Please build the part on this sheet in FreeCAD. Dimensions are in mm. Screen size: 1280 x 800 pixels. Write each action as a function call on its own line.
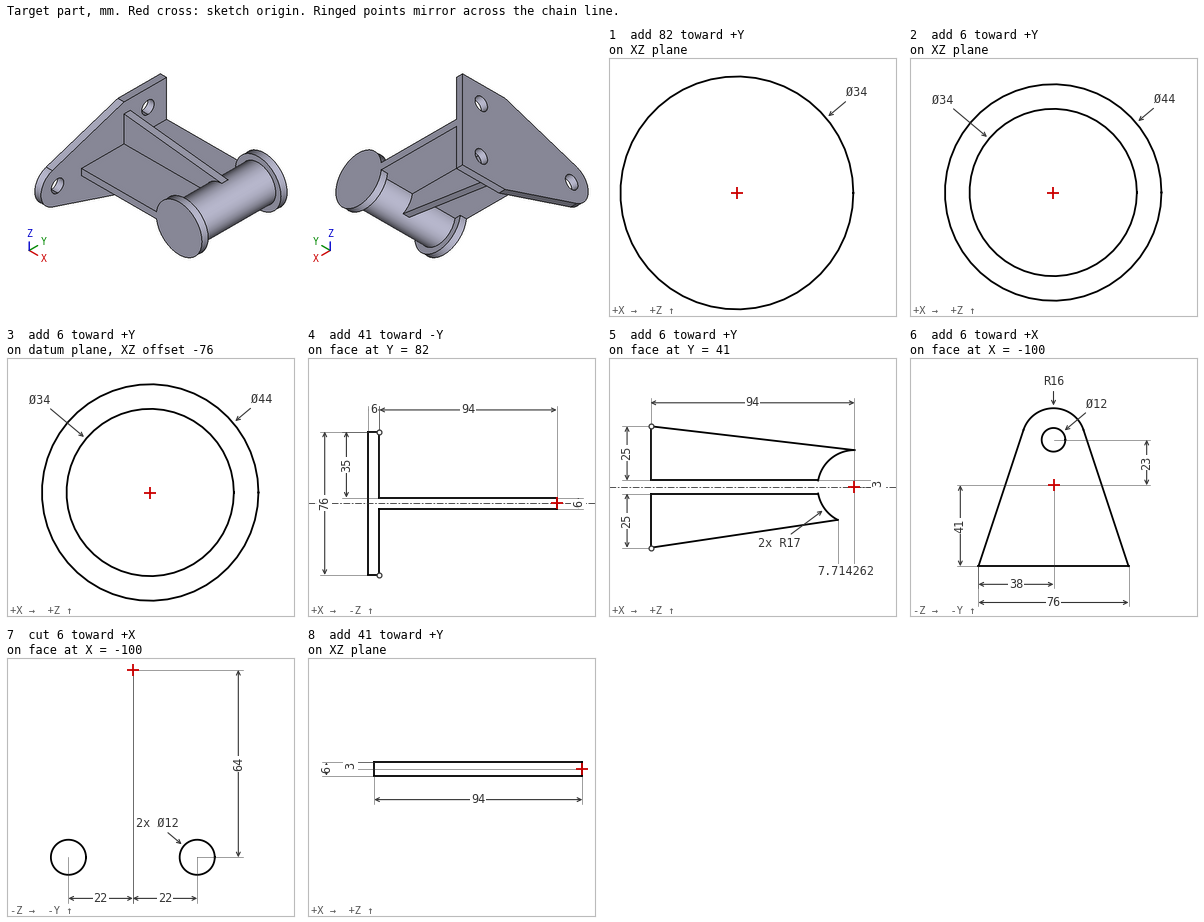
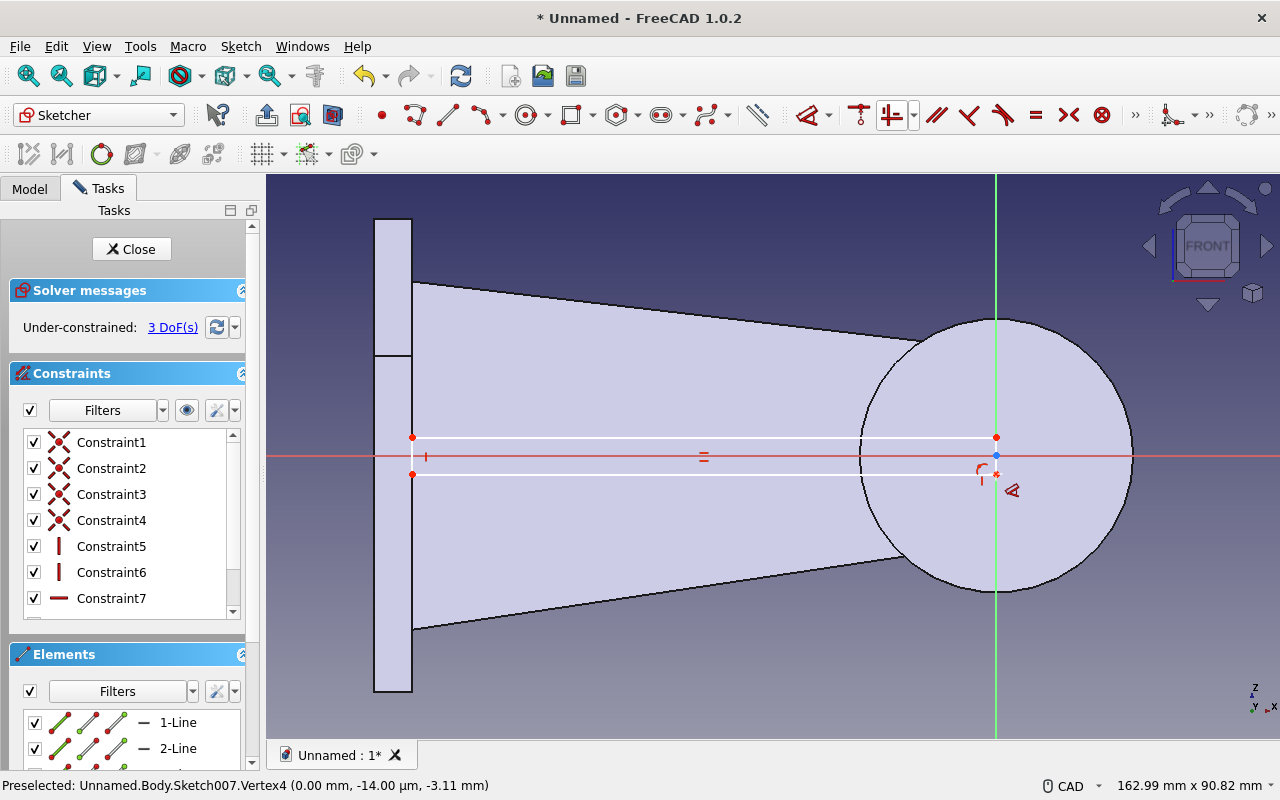
click(412, 453)
click(378, 469)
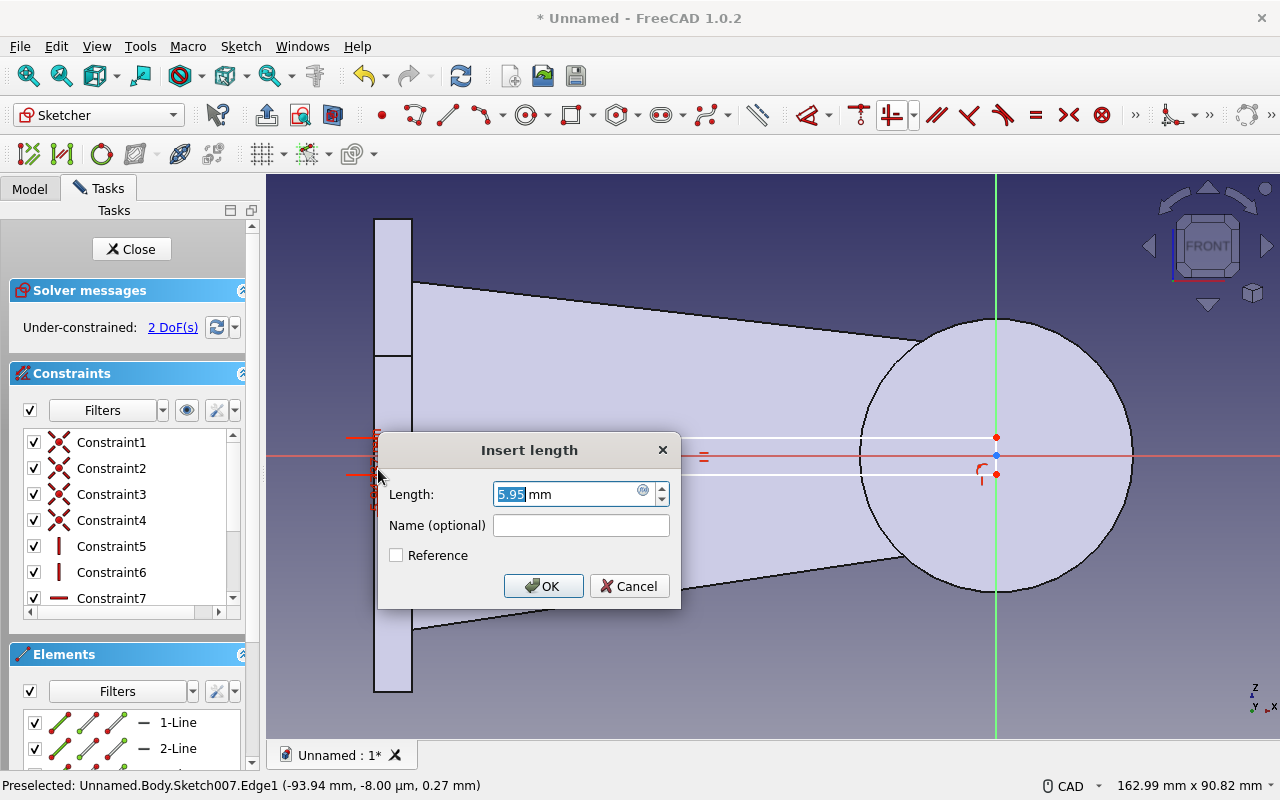
text(6)
key(Return)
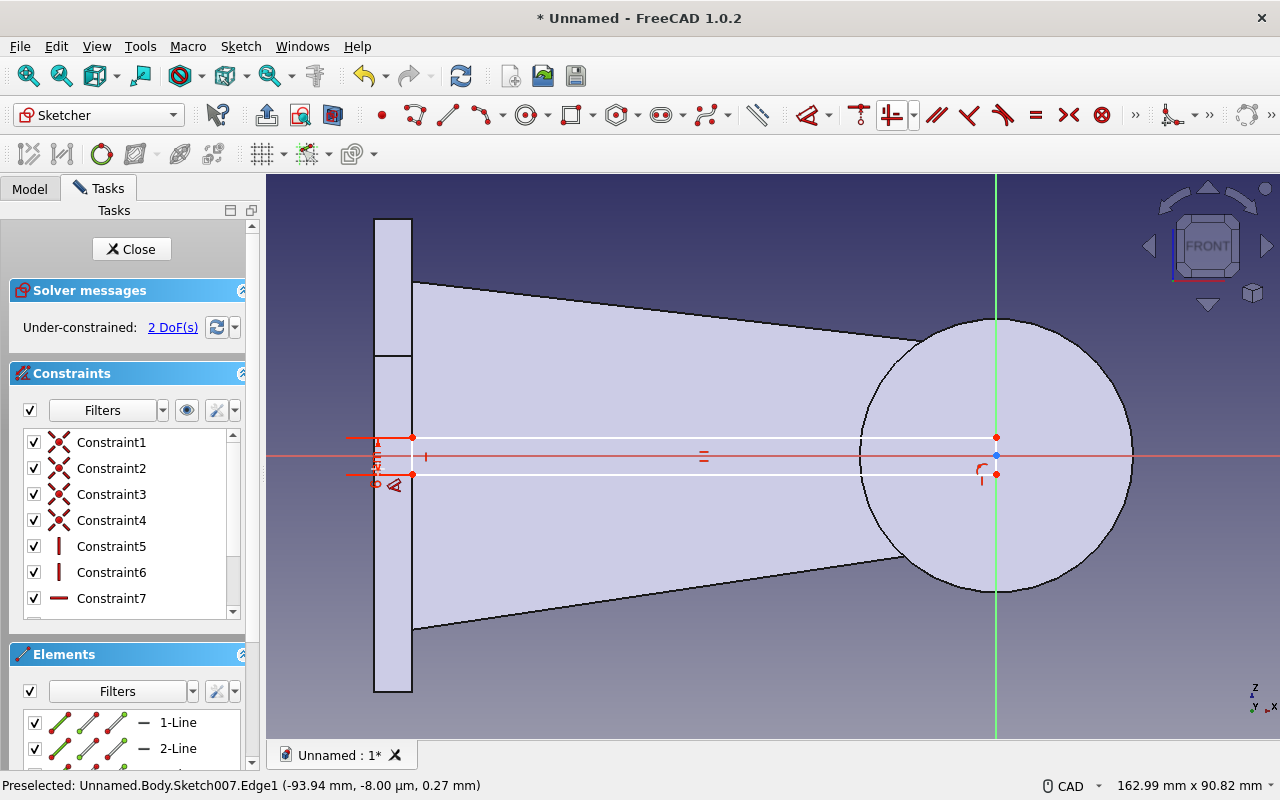
click(587, 475)
click(704, 509)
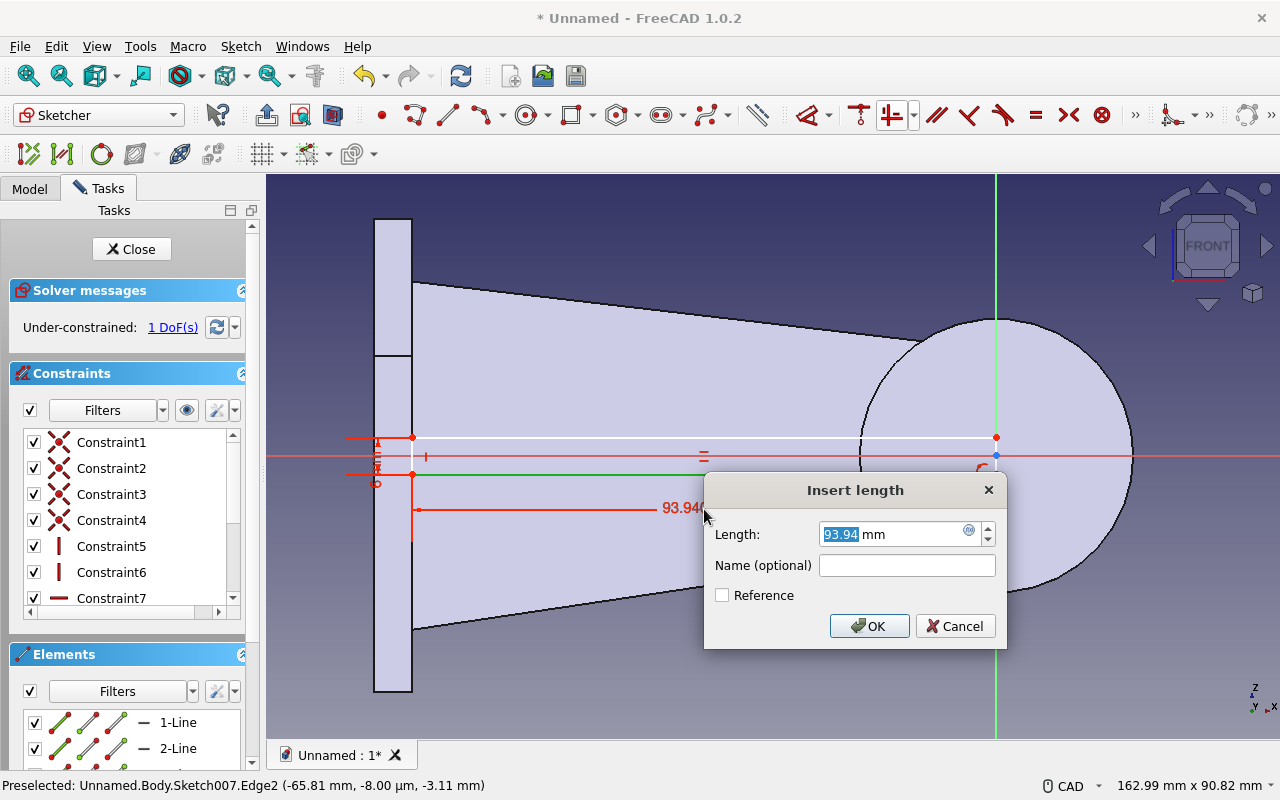
text(94)
key(Return)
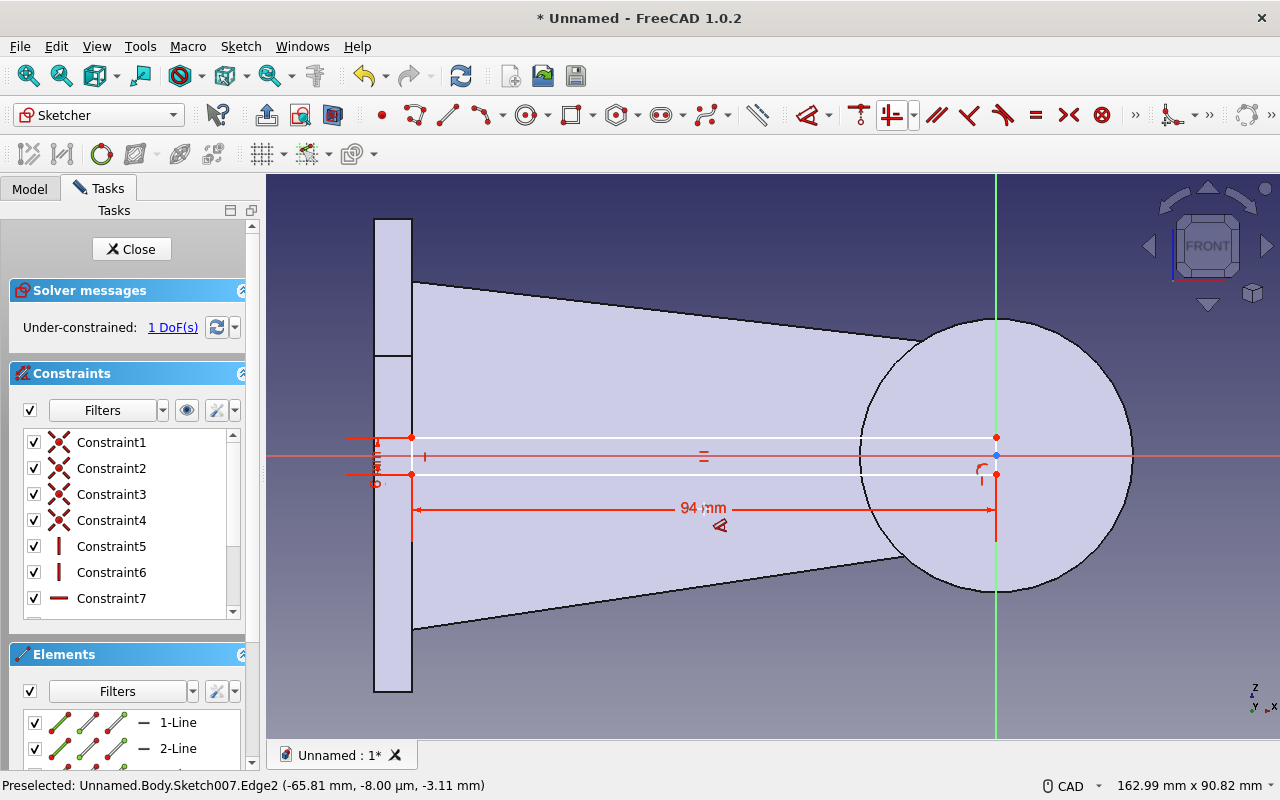
scroll(412, 438, up, 4)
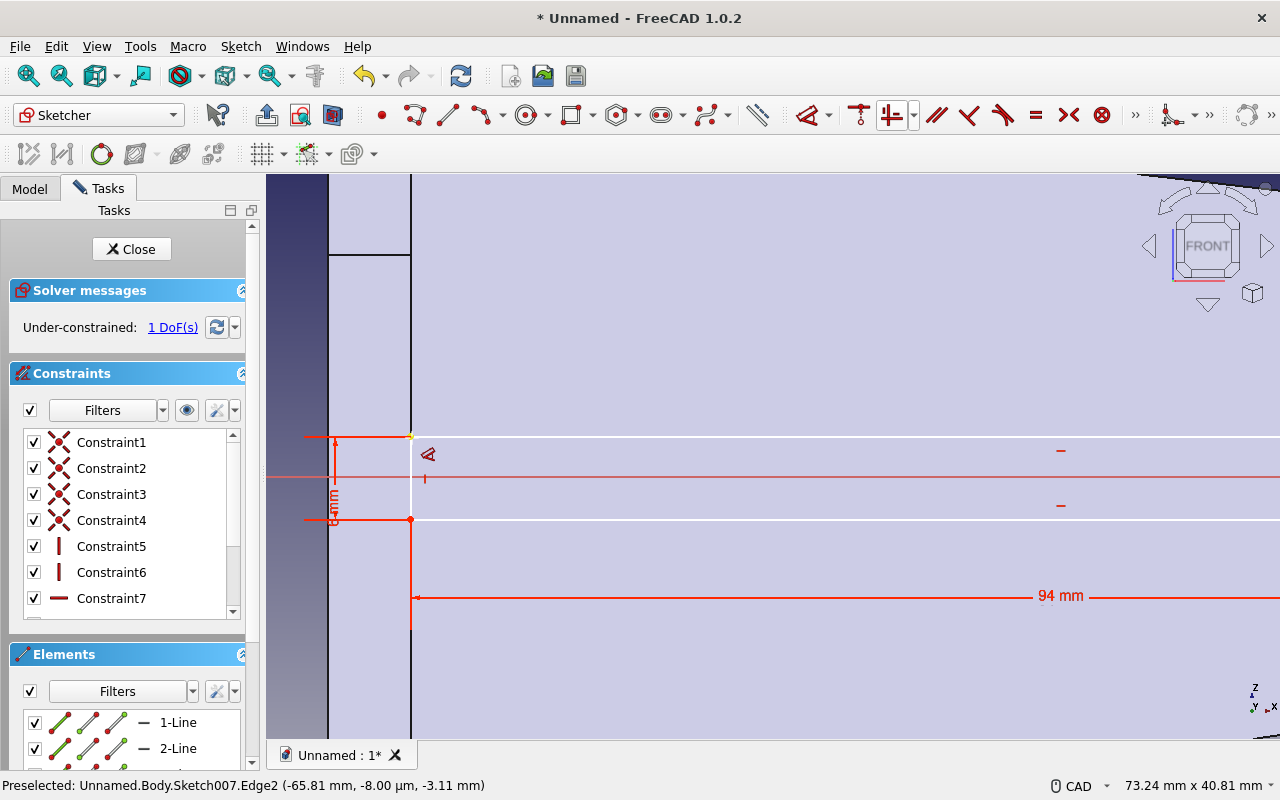
click(411, 437)
click(377, 457)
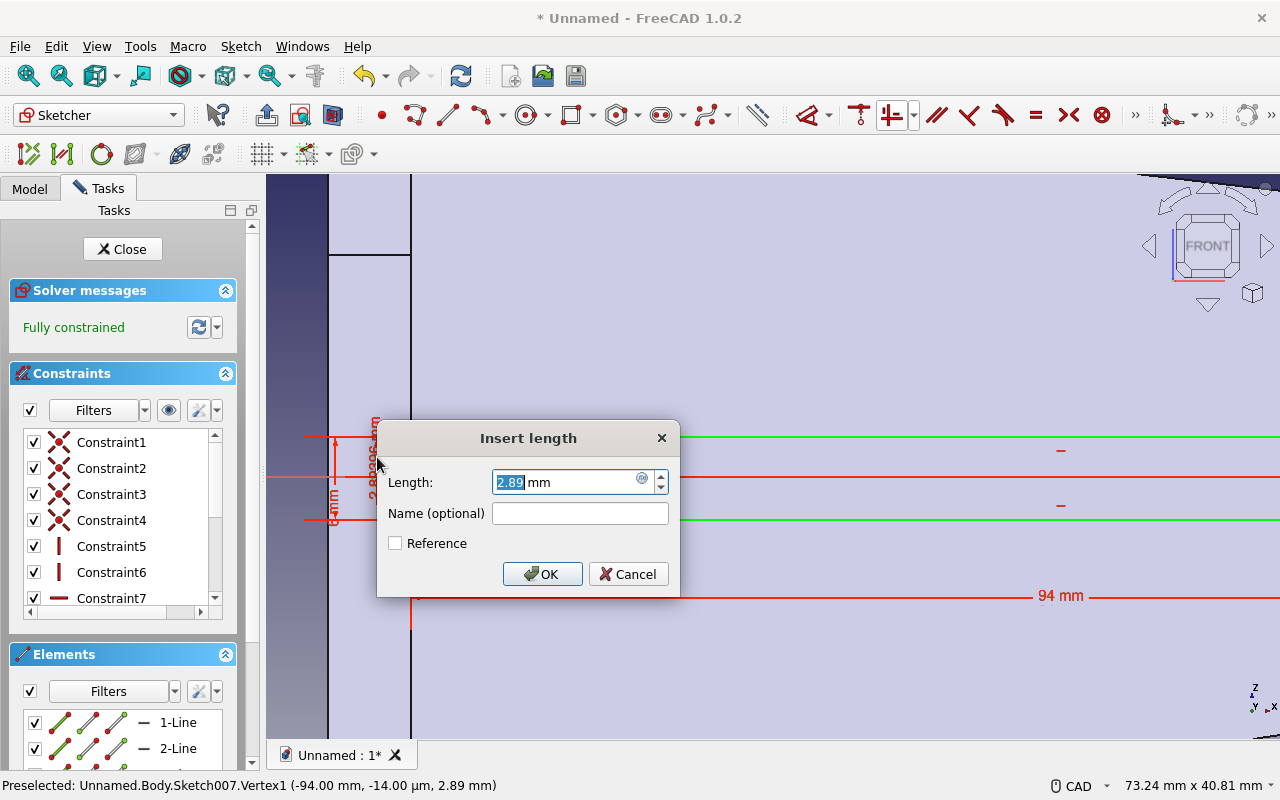
text(3)
key(Return)
key(Escape)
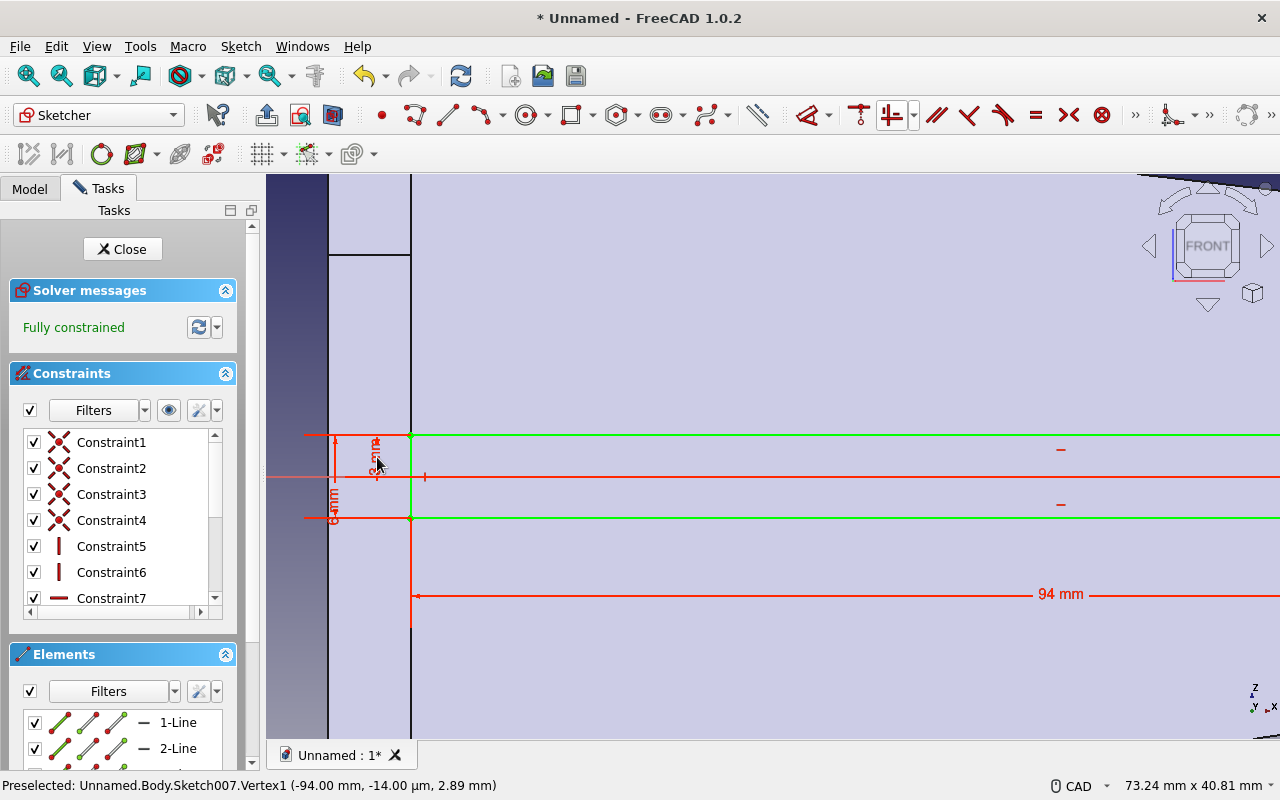
click(123, 249)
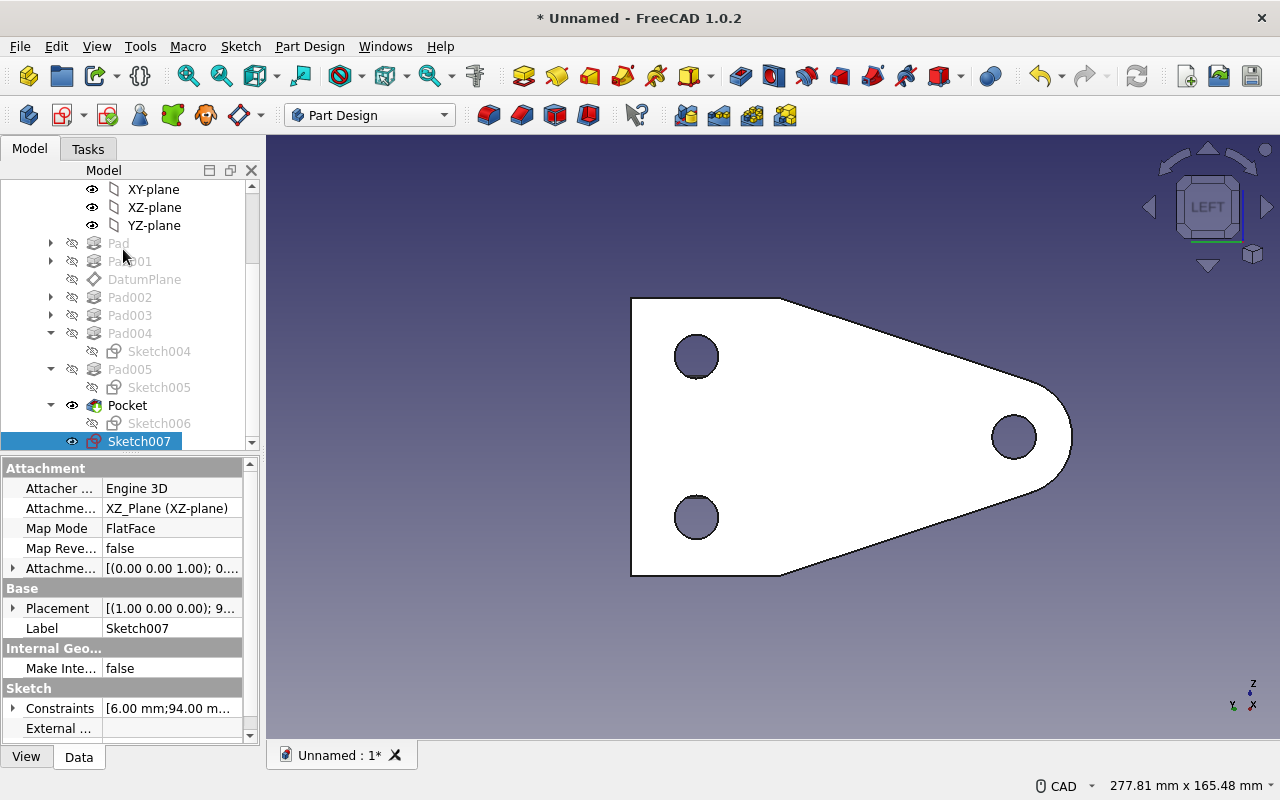
click(524, 76)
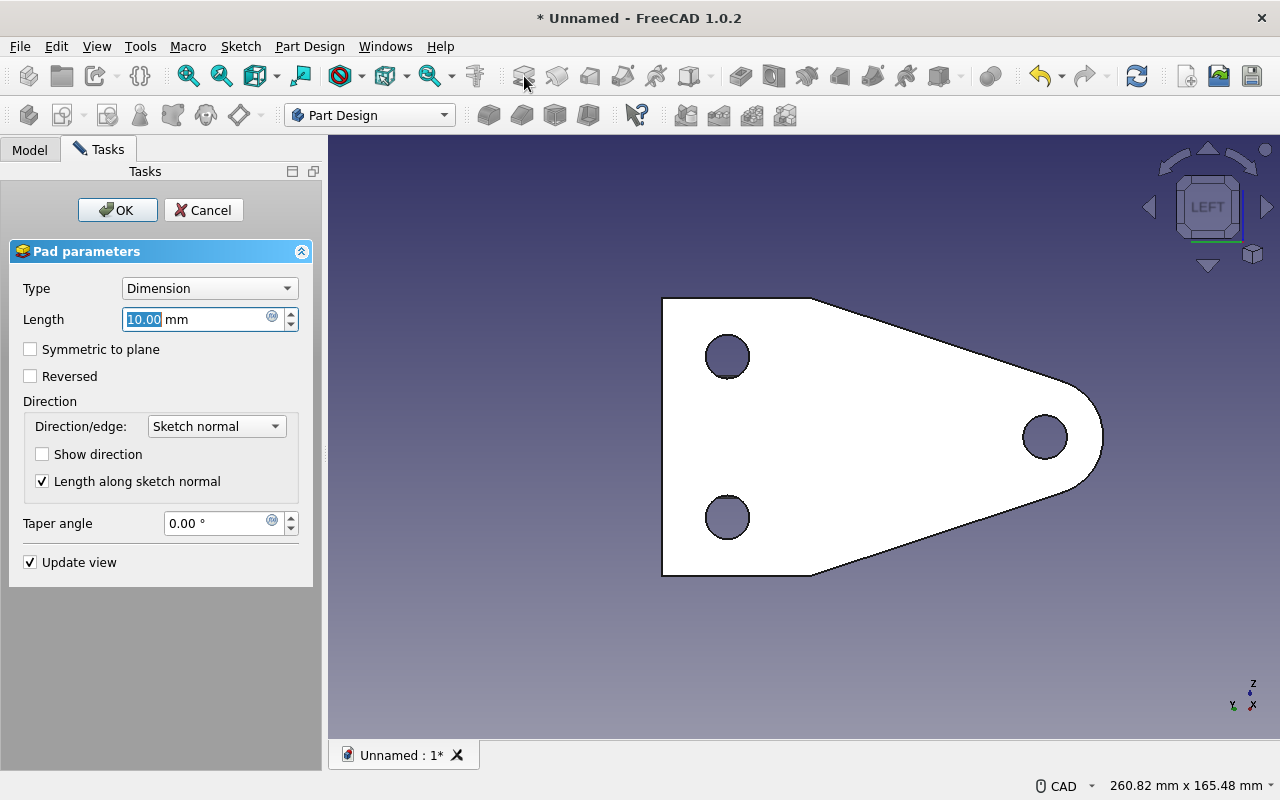
text(41)
key(Tab)